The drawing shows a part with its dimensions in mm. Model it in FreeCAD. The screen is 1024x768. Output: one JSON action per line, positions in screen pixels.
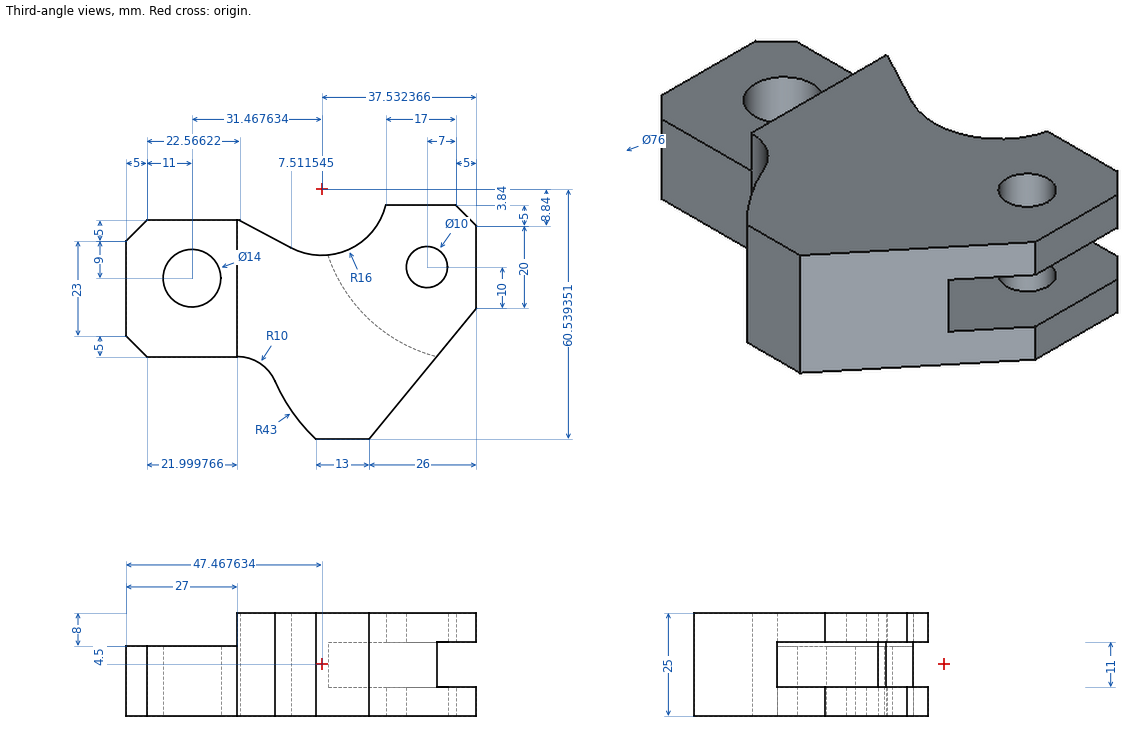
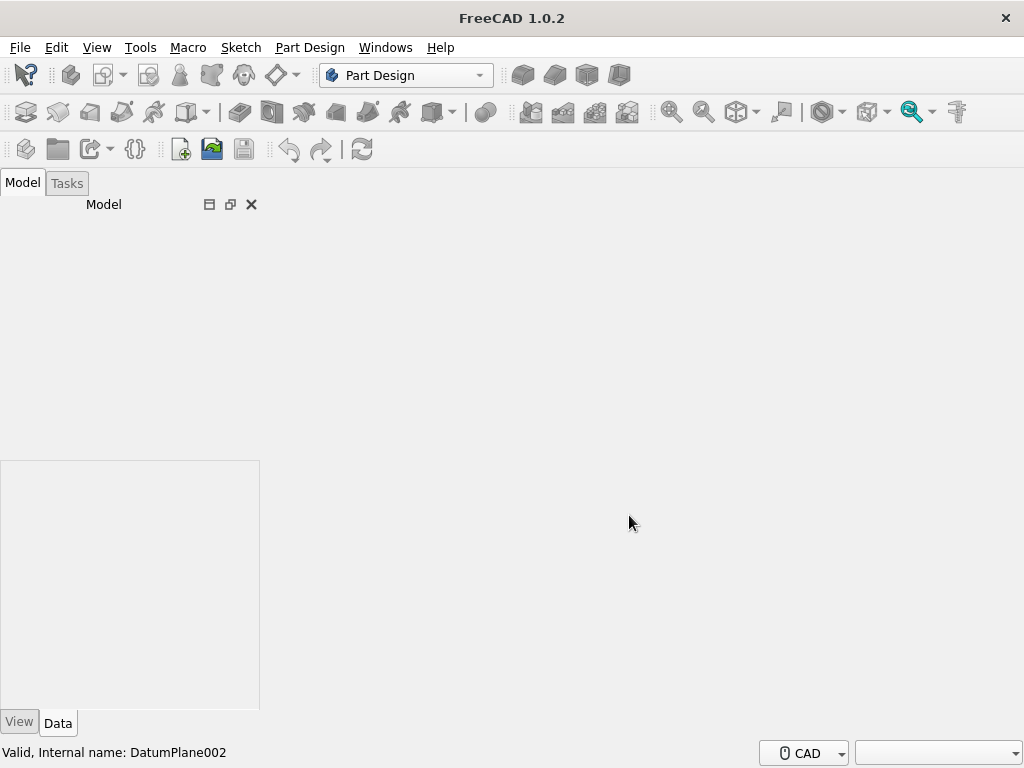
{"action": "left_click", "coordinate": [180, 150]}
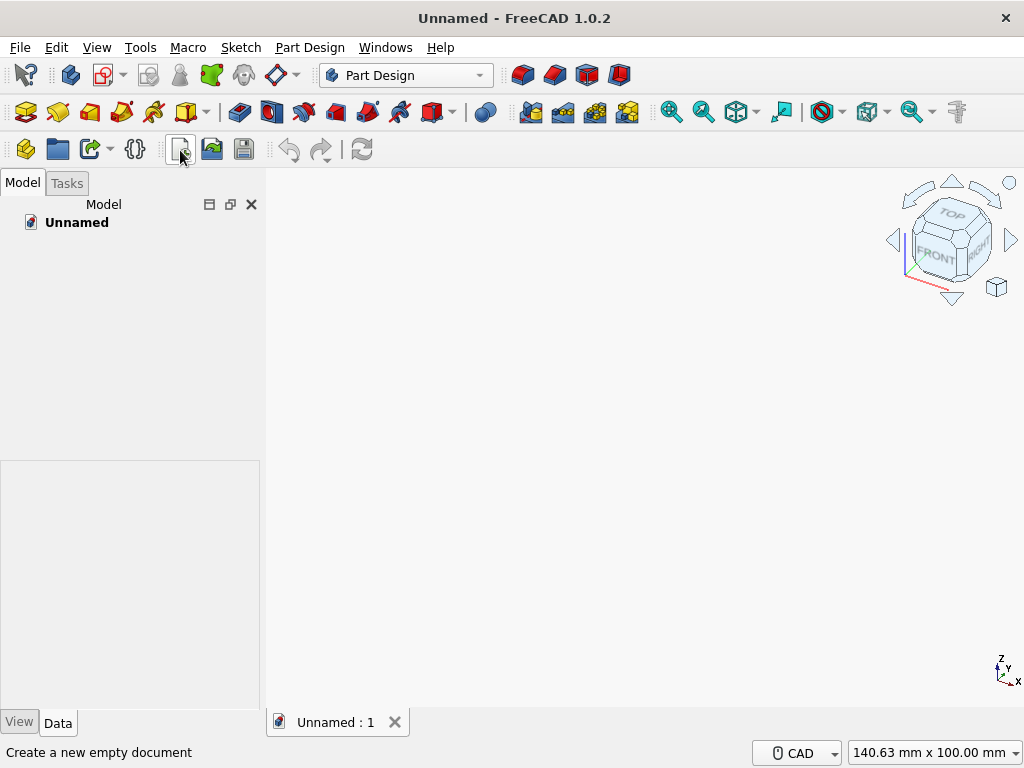
{"action": "left_click", "coordinate": [104, 76]}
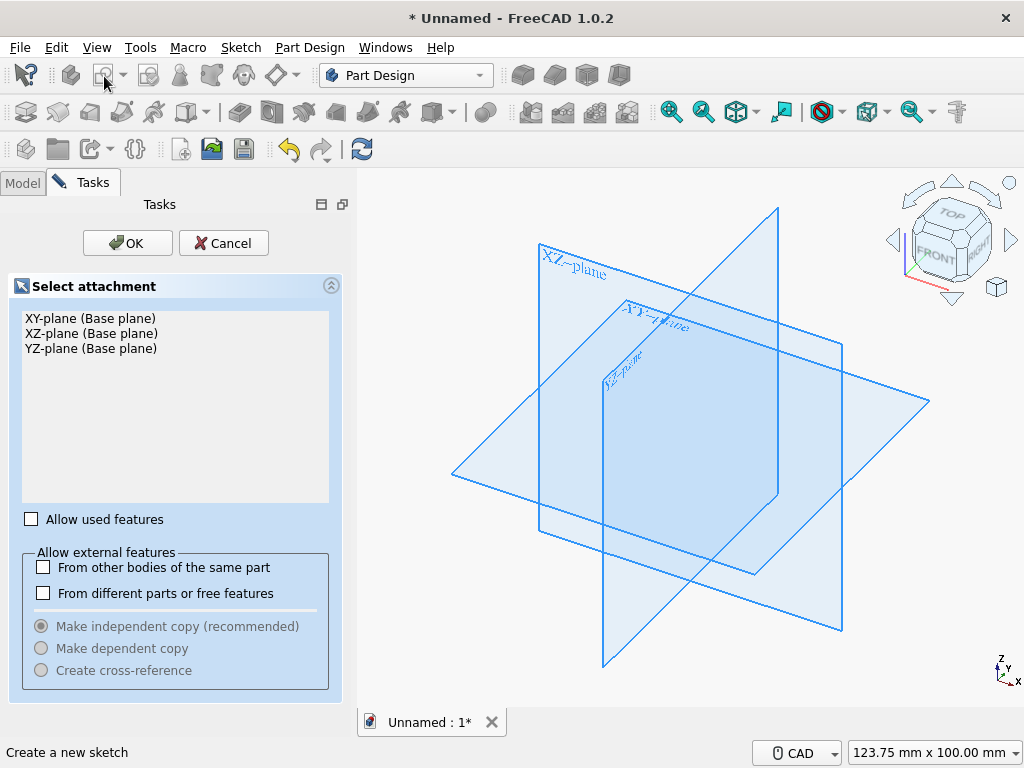
{"action": "left_click", "coordinate": [82, 318]}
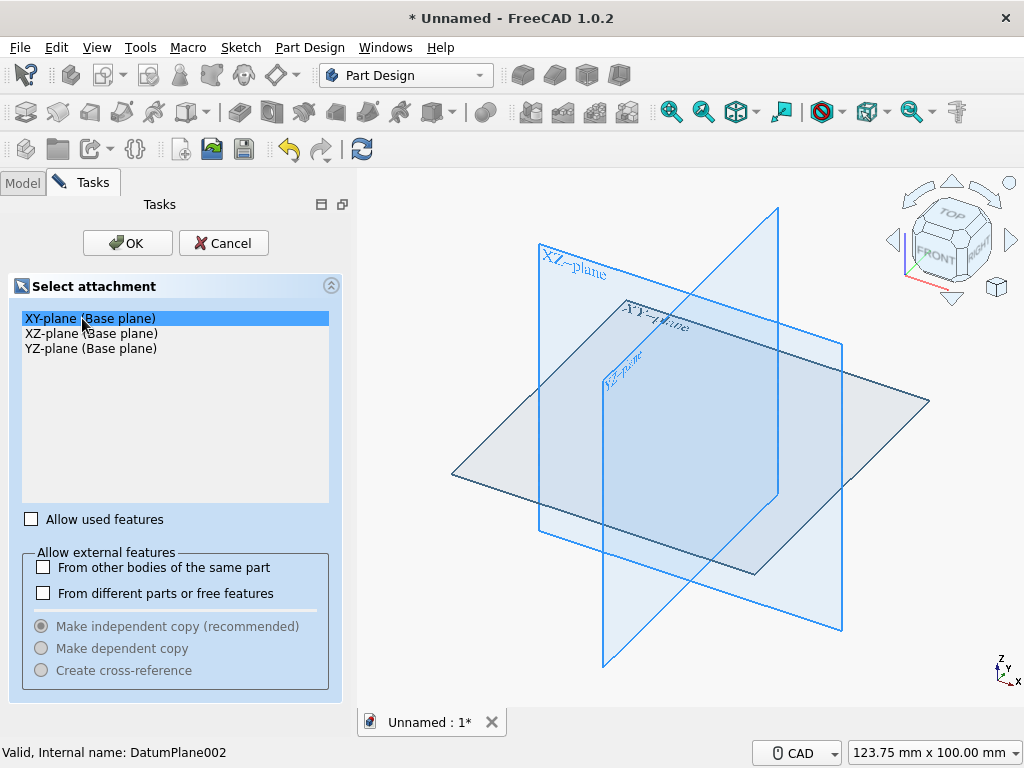
{"action": "left_click", "coordinate": [128, 243]}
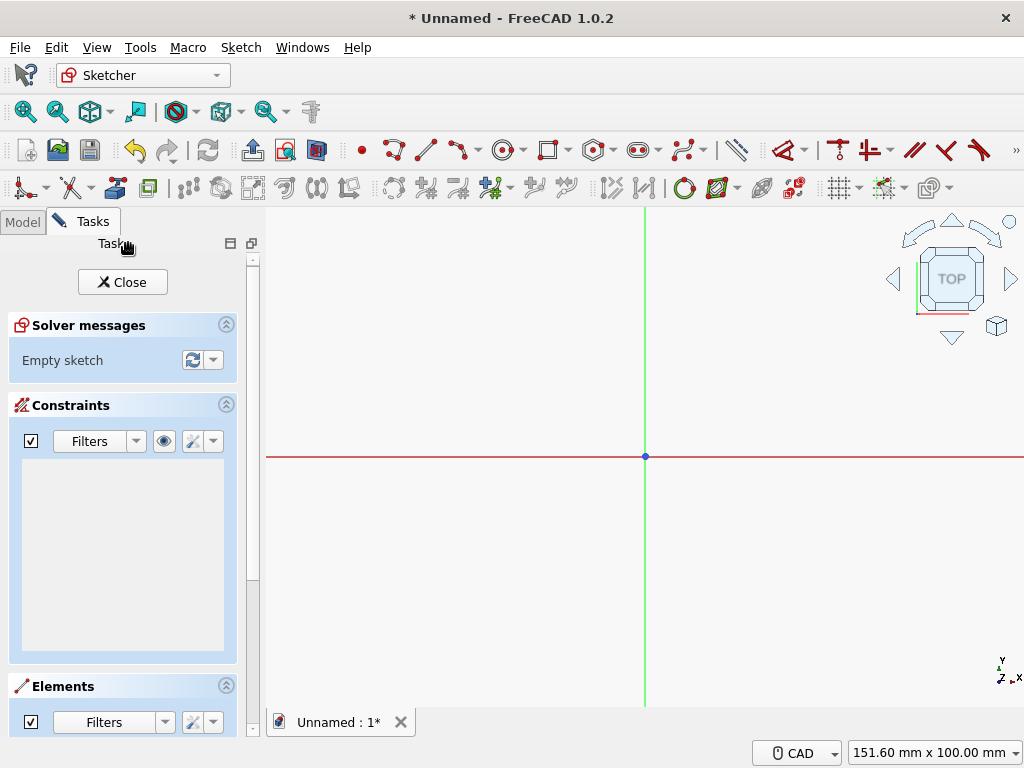
{"action": "scroll", "coordinate": [488, 235], "scroll_direction": "down", "scroll_amount": 2}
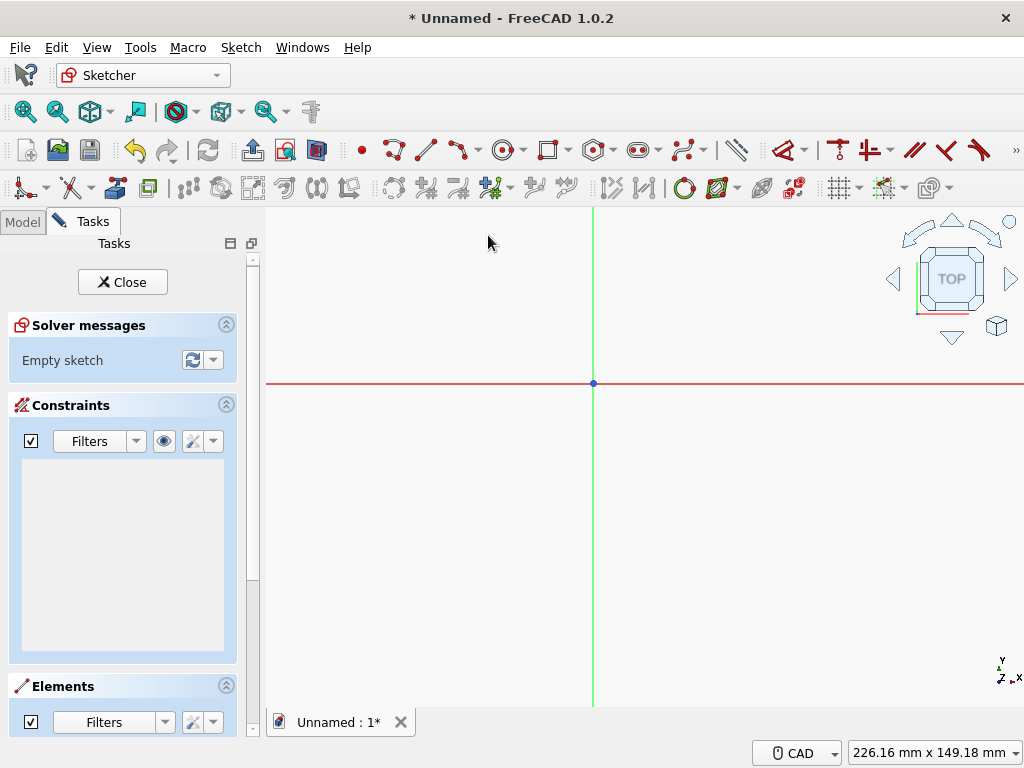
{"action": "scroll", "coordinate": [577, 543], "scroll_direction": "up", "scroll_amount": 2}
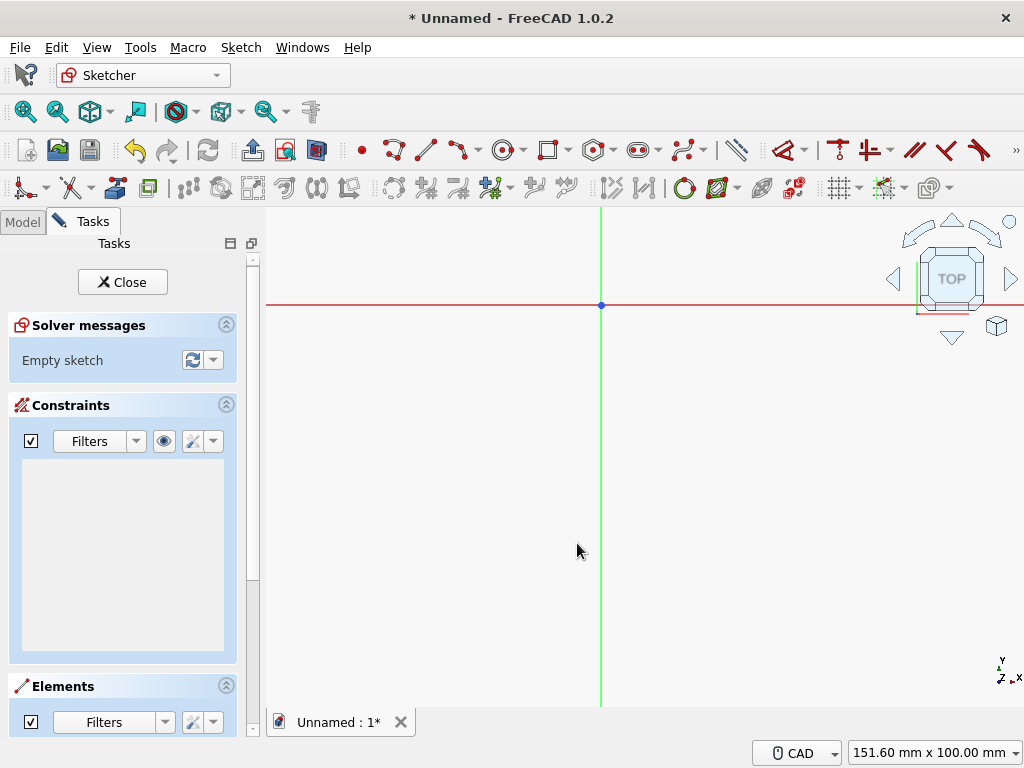
{"action": "left_click", "coordinate": [394, 150]}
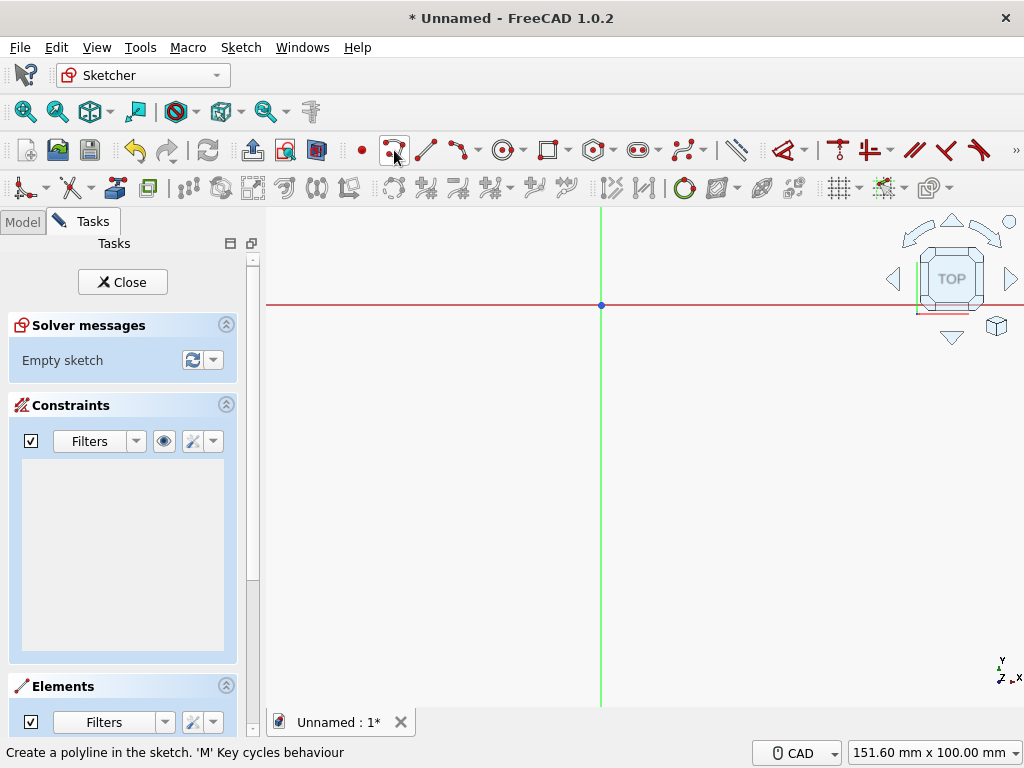
{"action": "scroll", "coordinate": [594, 608], "scroll_direction": "up", "scroll_amount": 4}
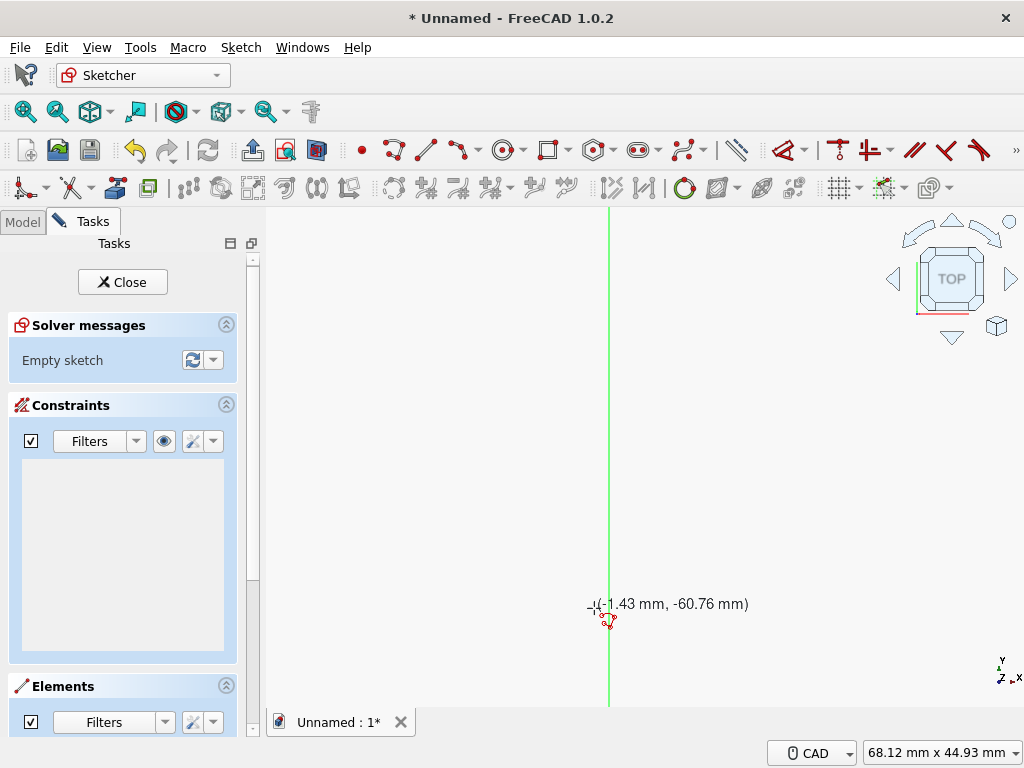
{"action": "left_click", "coordinate": [593, 607]}
{"action": "left_click", "coordinate": [738, 607]}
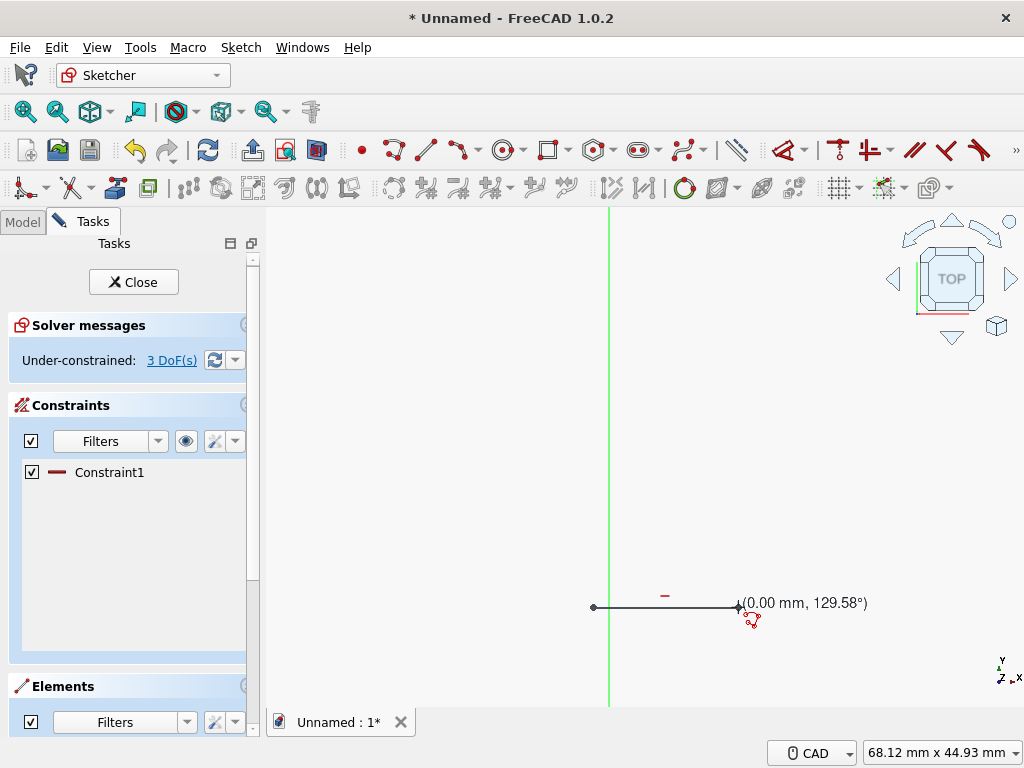
{"action": "scroll", "coordinate": [595, 610], "scroll_direction": "down", "scroll_amount": 4}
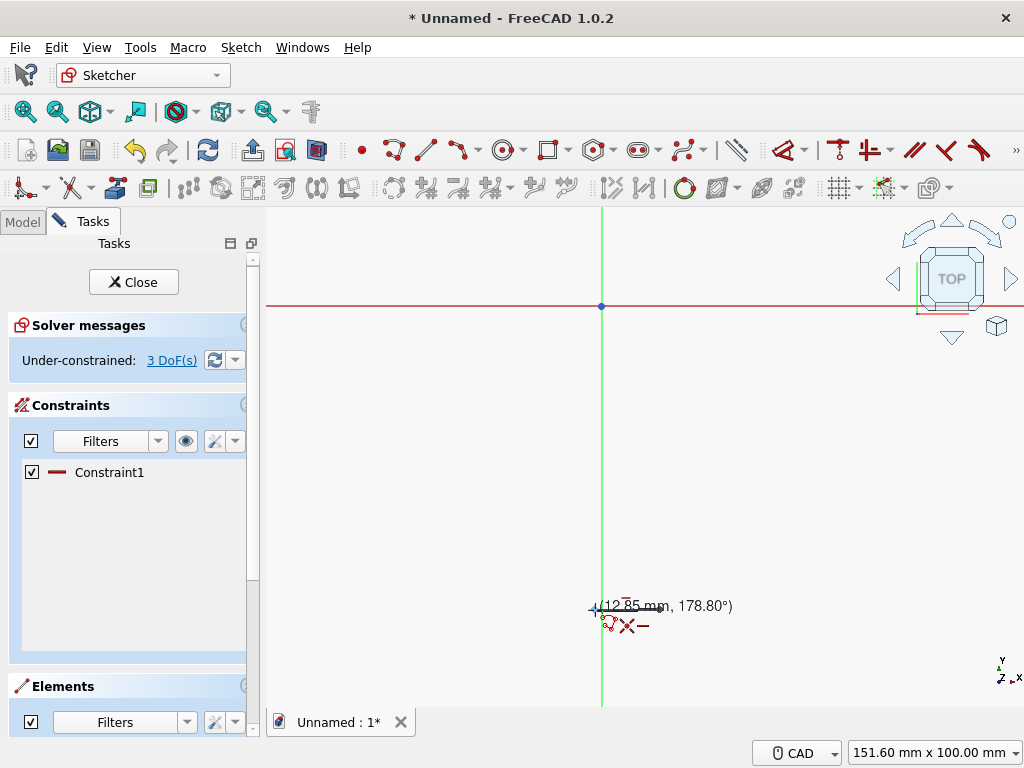
{"action": "left_click", "coordinate": [789, 451]}
{"action": "left_click", "coordinate": [789, 351]}
{"action": "left_click", "coordinate": [764, 326]}
{"action": "left_click", "coordinate": [679, 326]}
{"action": "right_click", "coordinate": [679, 326]}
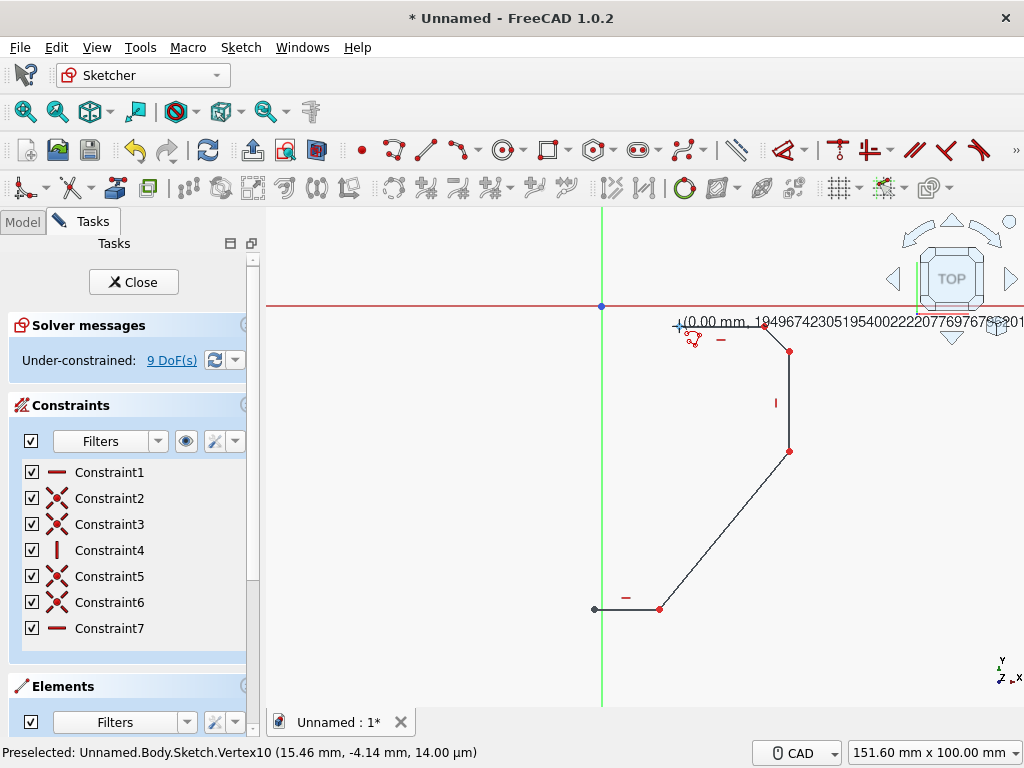
{"action": "left_click", "coordinate": [564, 377]}
{"action": "left_click", "coordinate": [502, 344]}
{"action": "left_click", "coordinate": [389, 344]}
{"action": "left_click", "coordinate": [364, 369]}
{"action": "left_click", "coordinate": [364, 484]}
{"action": "left_click", "coordinate": [389, 509]}
{"action": "left_click", "coordinate": [499, 509]}
{"action": "right_click", "coordinate": [499, 509]}